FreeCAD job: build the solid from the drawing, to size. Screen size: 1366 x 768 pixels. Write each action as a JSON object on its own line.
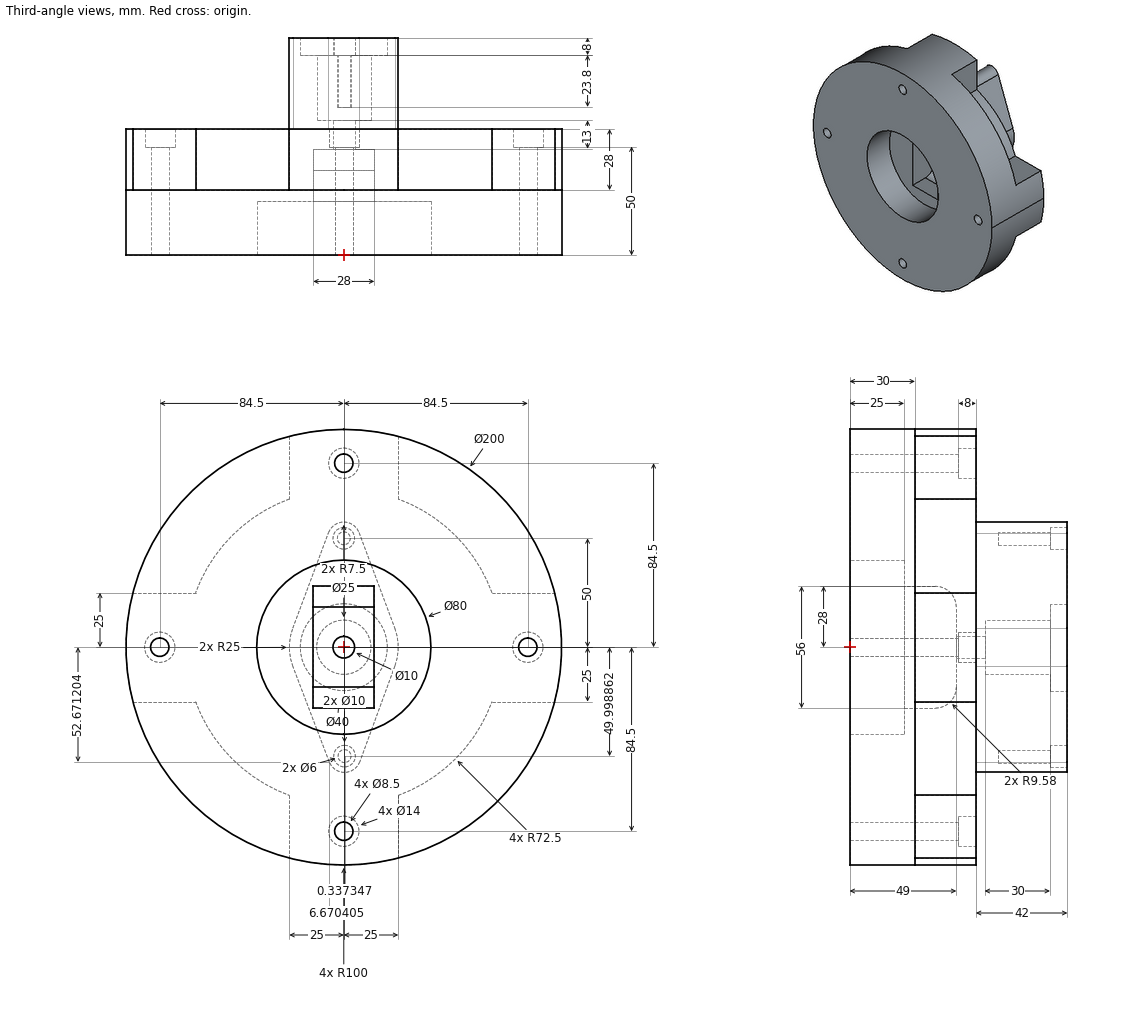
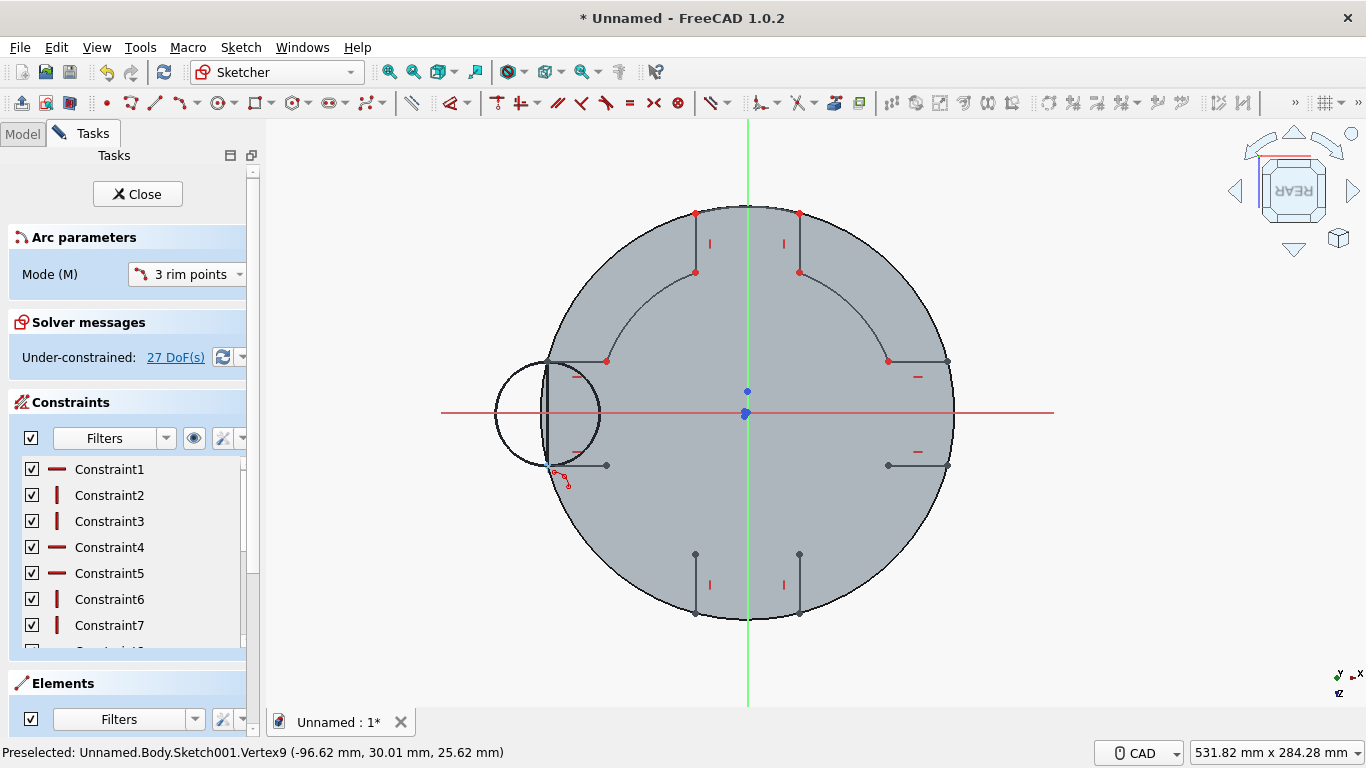
{"action": "scroll", "coordinate": [541, 403], "scroll_direction": "up", "scroll_amount": 5}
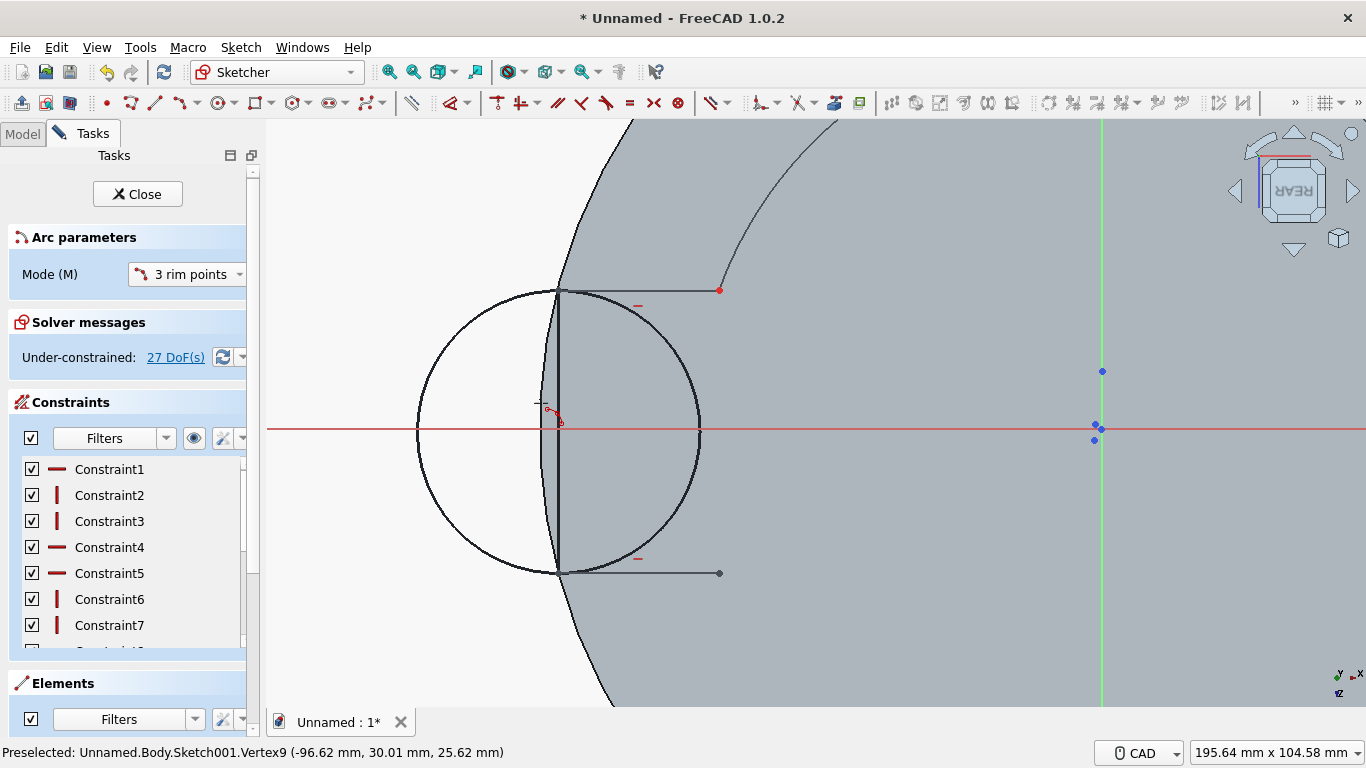
{"action": "left_click", "coordinate": [540, 401]}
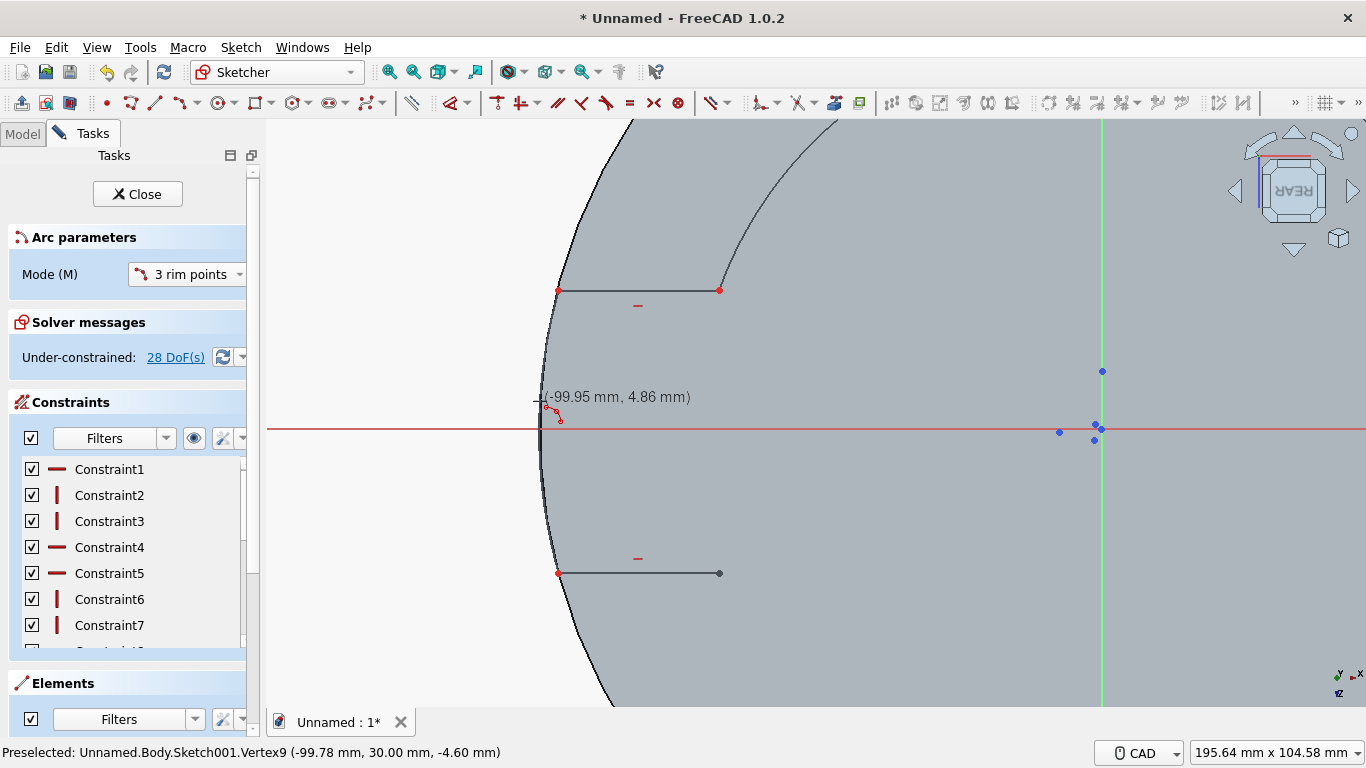
{"action": "left_click", "coordinate": [719, 573]}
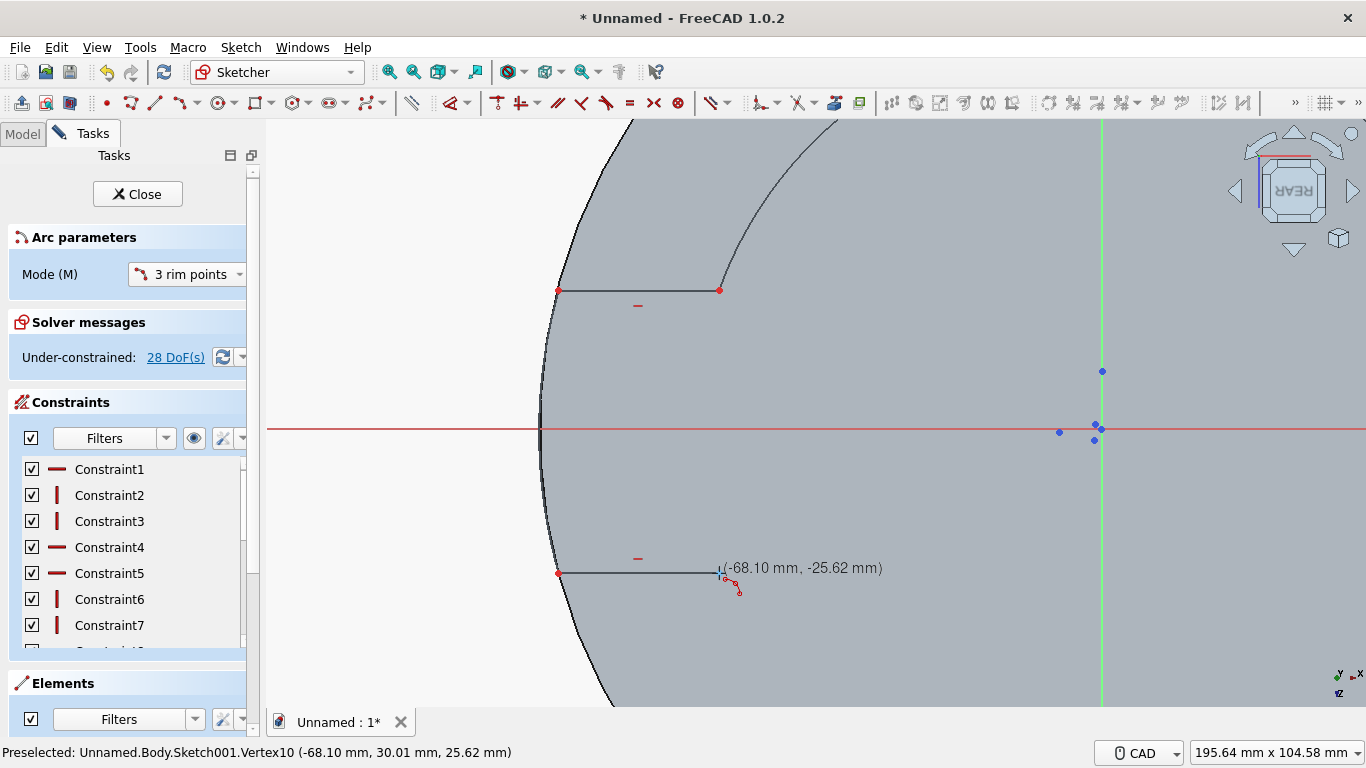
{"action": "scroll", "coordinate": [541, 403], "scroll_direction": "down", "scroll_amount": 5}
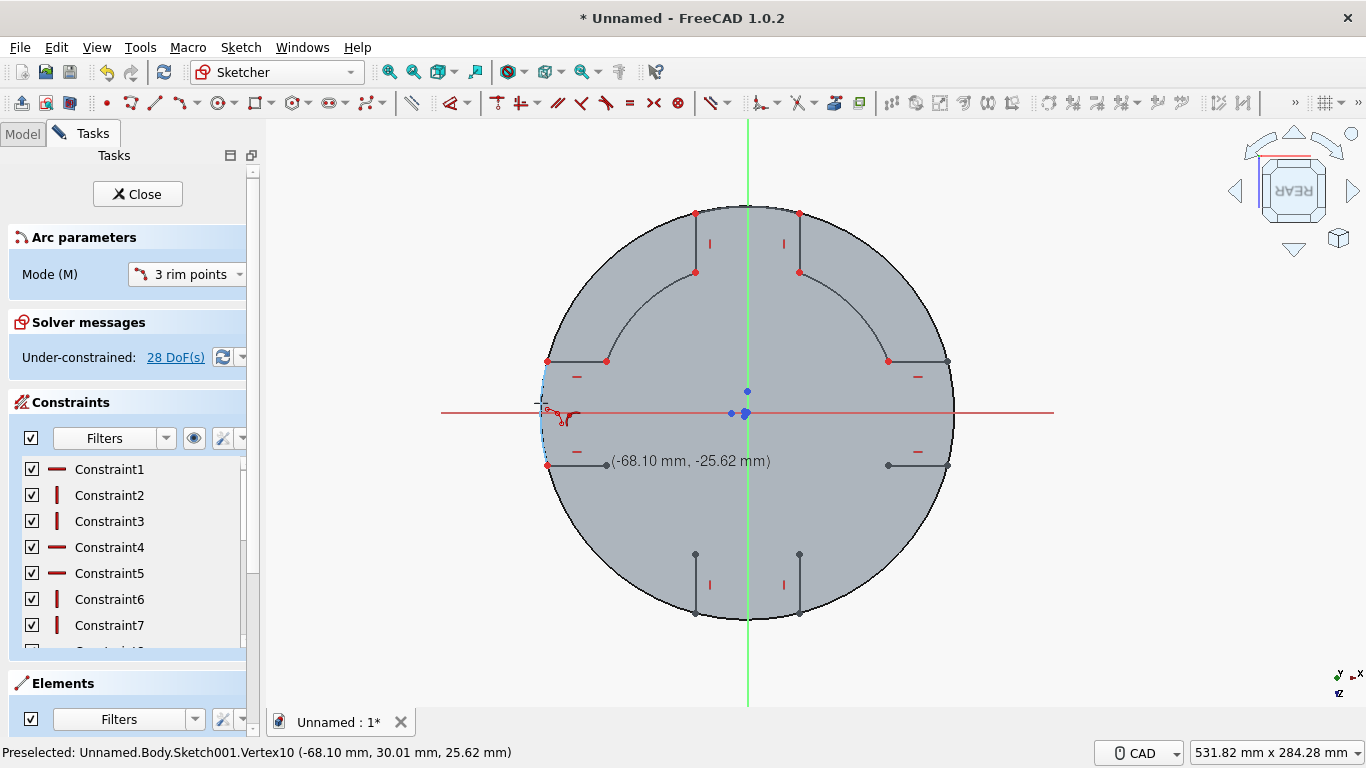
{"action": "left_click", "coordinate": [696, 555]}
{"action": "left_click", "coordinate": [641, 519]}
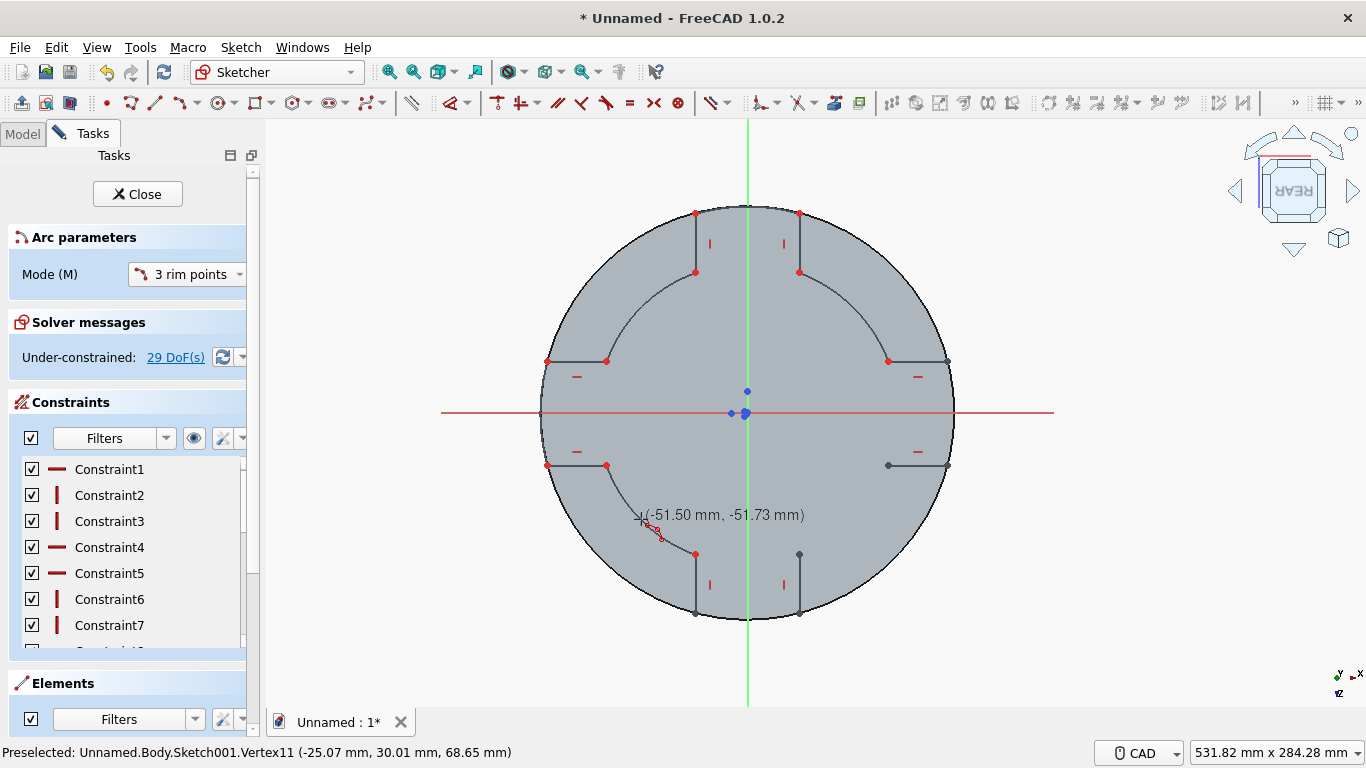
{"action": "left_click", "coordinate": [696, 614]}
{"action": "left_click", "coordinate": [800, 614]}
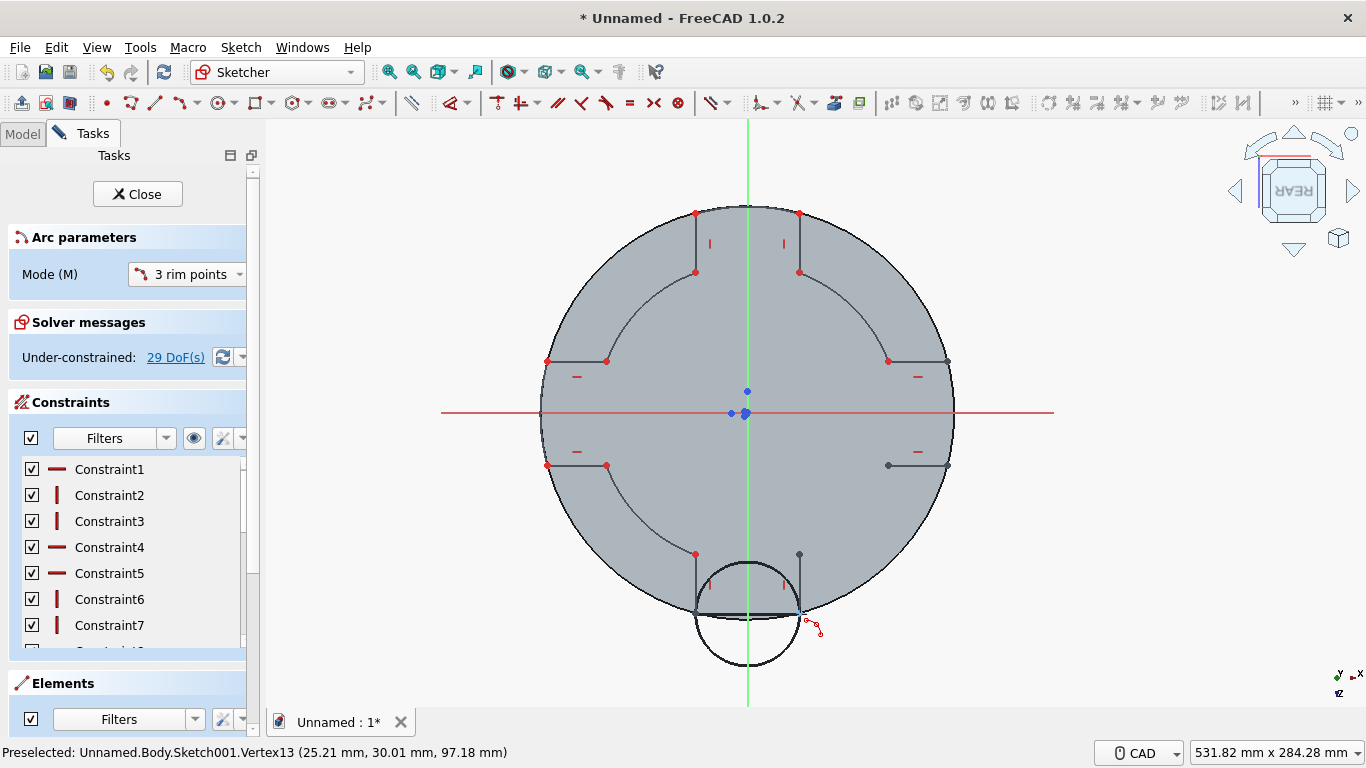
{"action": "scroll", "coordinate": [737, 620], "scroll_direction": "up", "scroll_amount": 5}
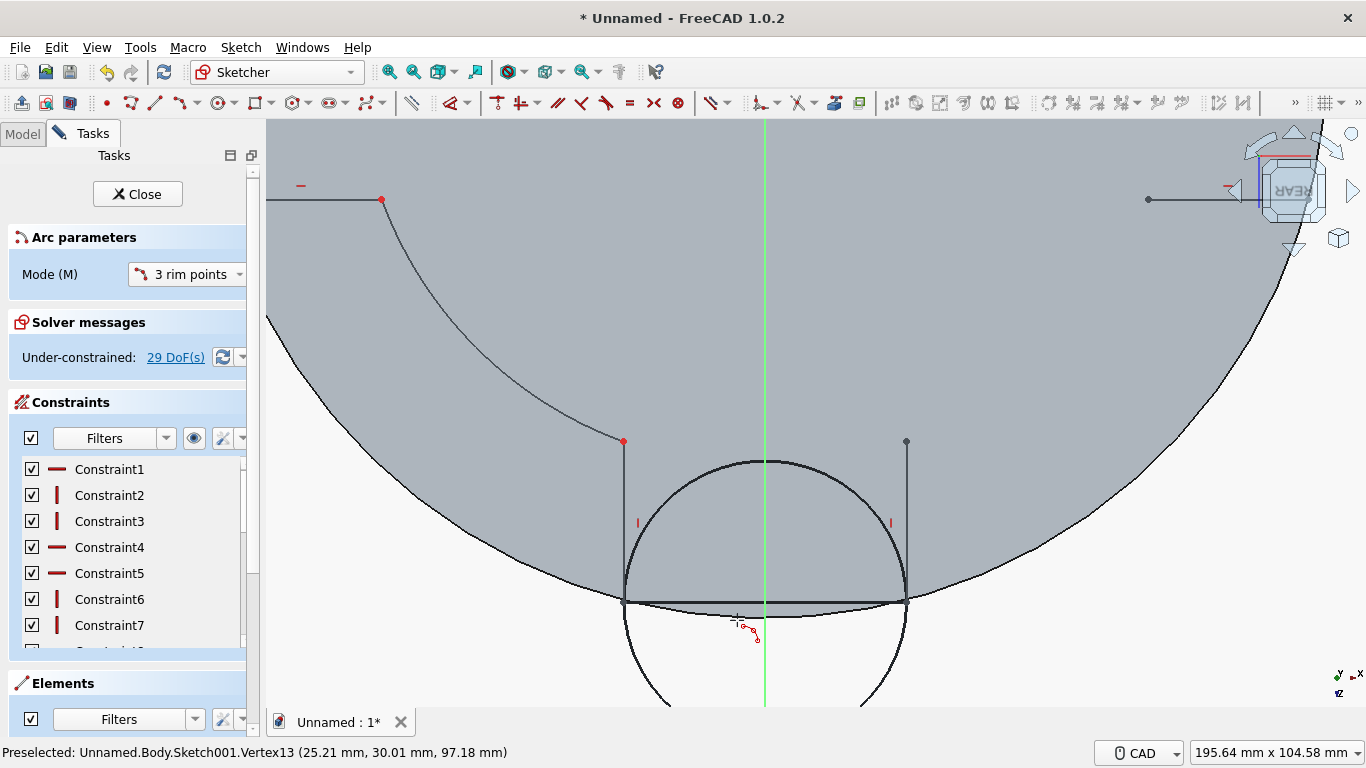
{"action": "left_click", "coordinate": [736, 617]}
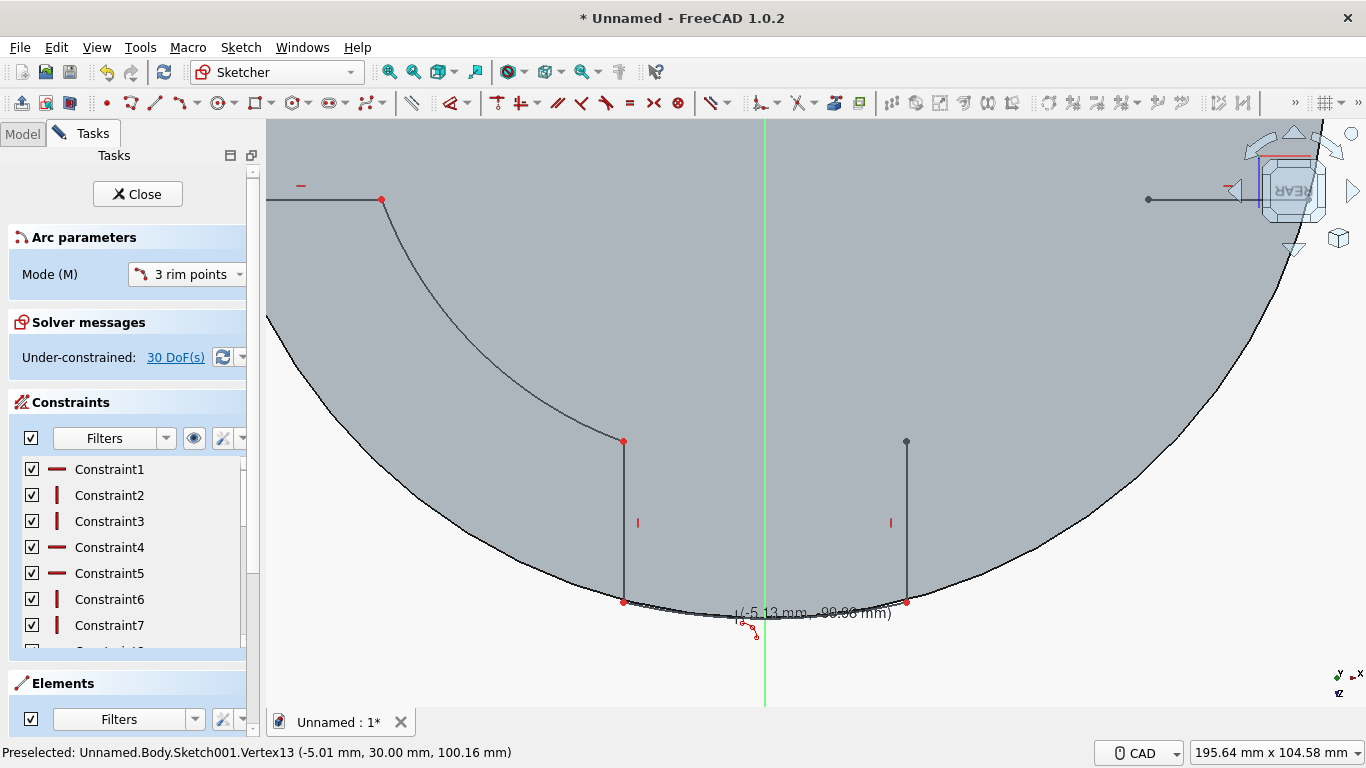
{"action": "left_click", "coordinate": [907, 442]}
{"action": "left_click", "coordinate": [1149, 200]}
{"action": "left_click", "coordinate": [1053, 344]}